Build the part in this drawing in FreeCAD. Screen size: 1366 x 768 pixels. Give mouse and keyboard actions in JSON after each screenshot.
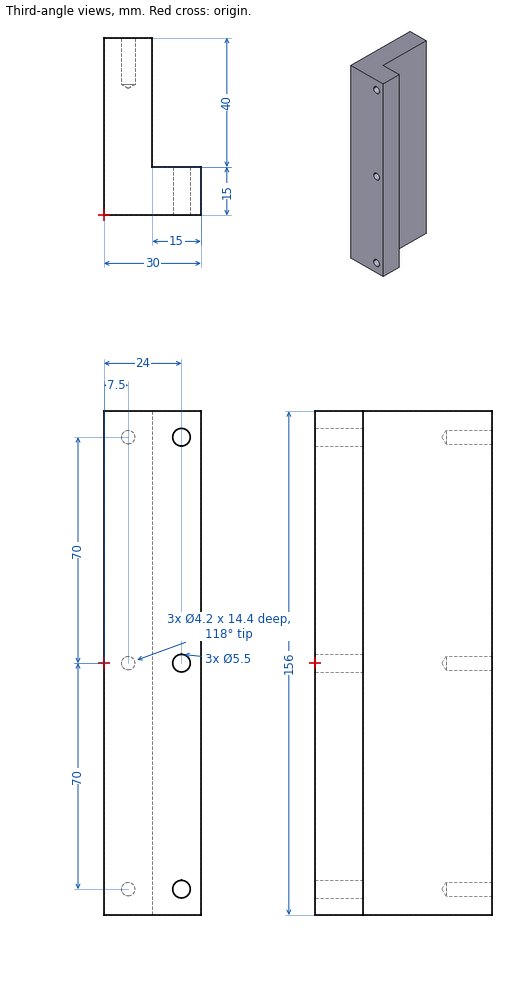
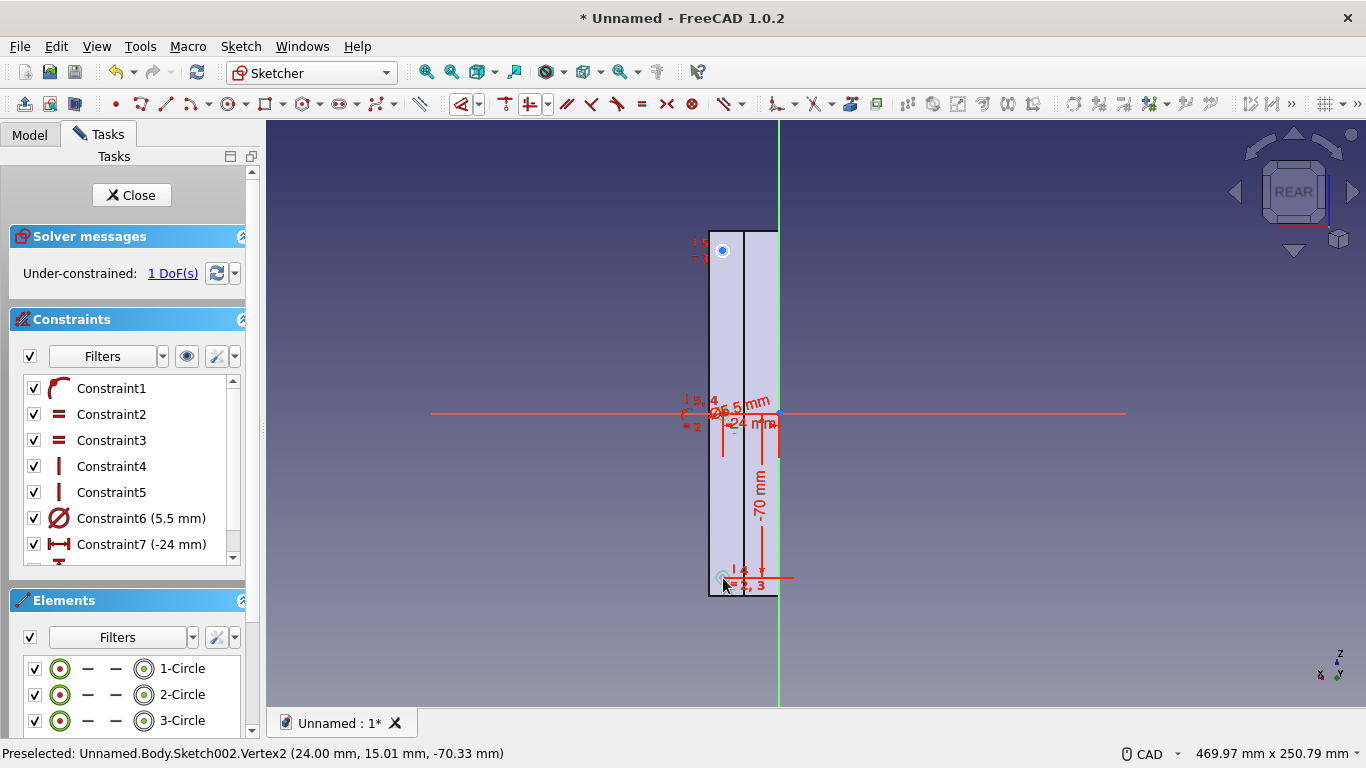
{"action": "left_click", "coordinate": [723, 251]}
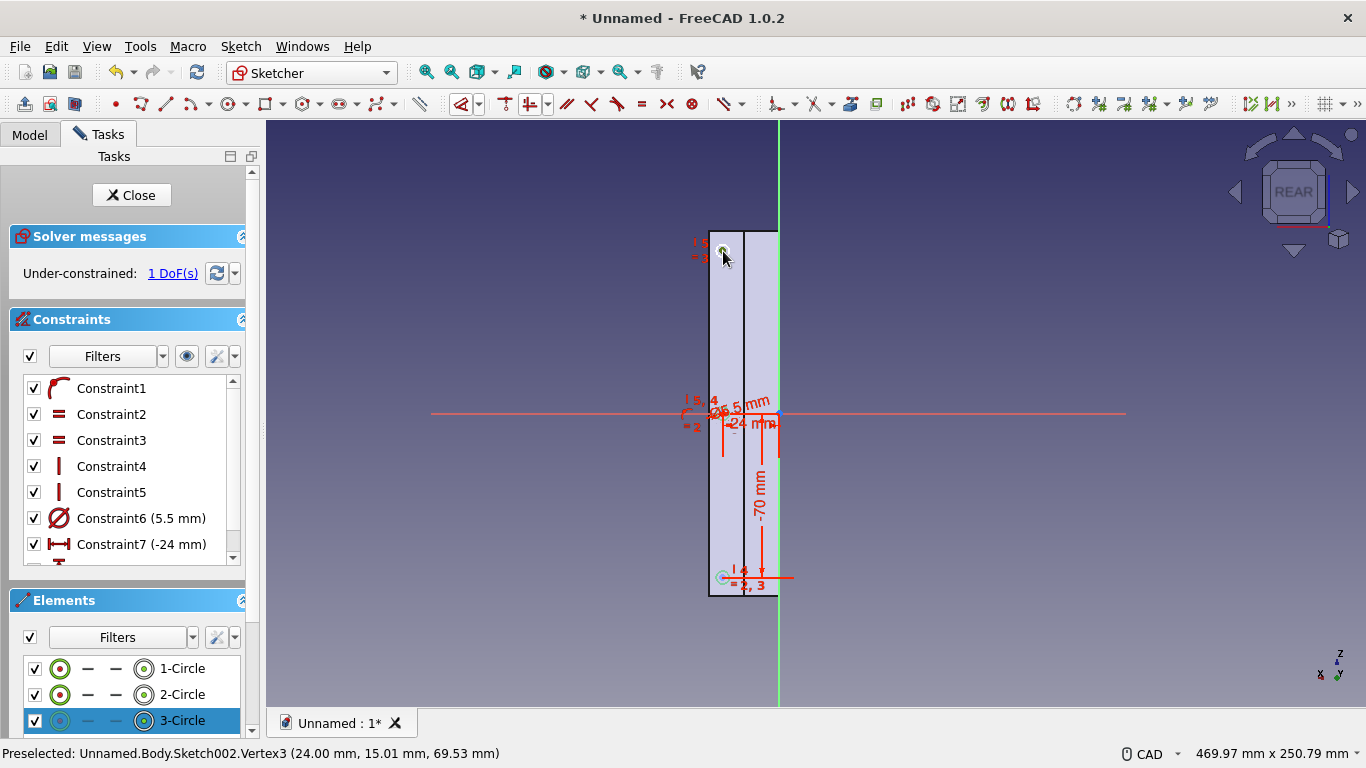
{"action": "key", "text": "i"}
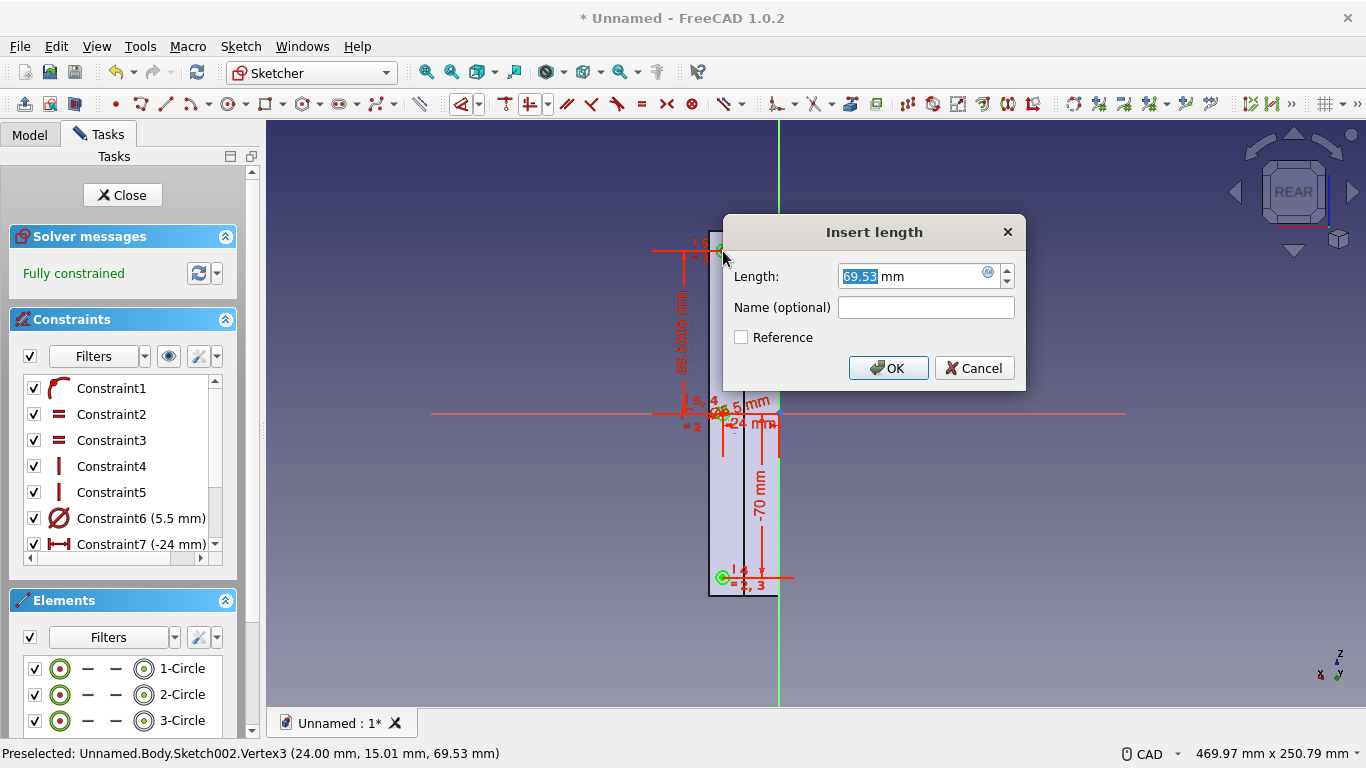
{"action": "type", "text": "70"}
{"action": "key", "text": "Return"}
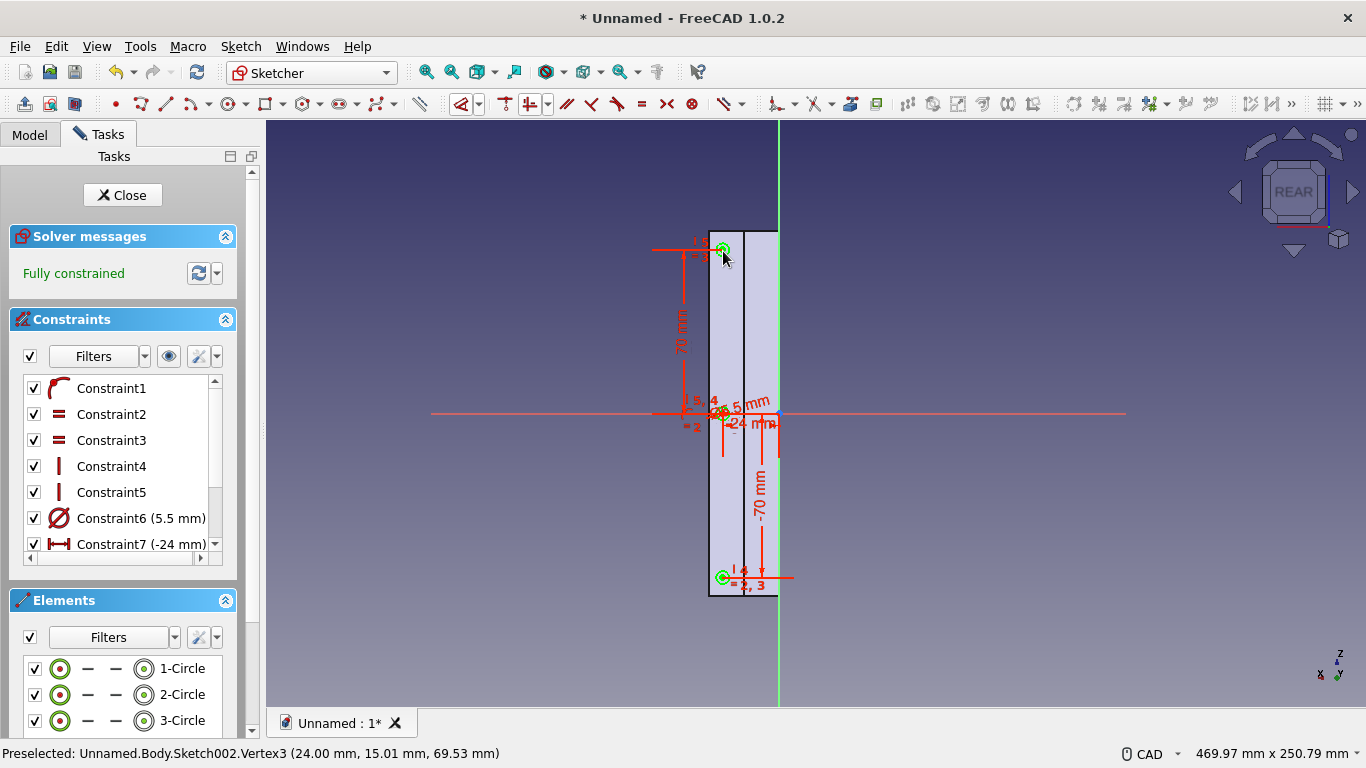
{"action": "left_click", "coordinate": [123, 195]}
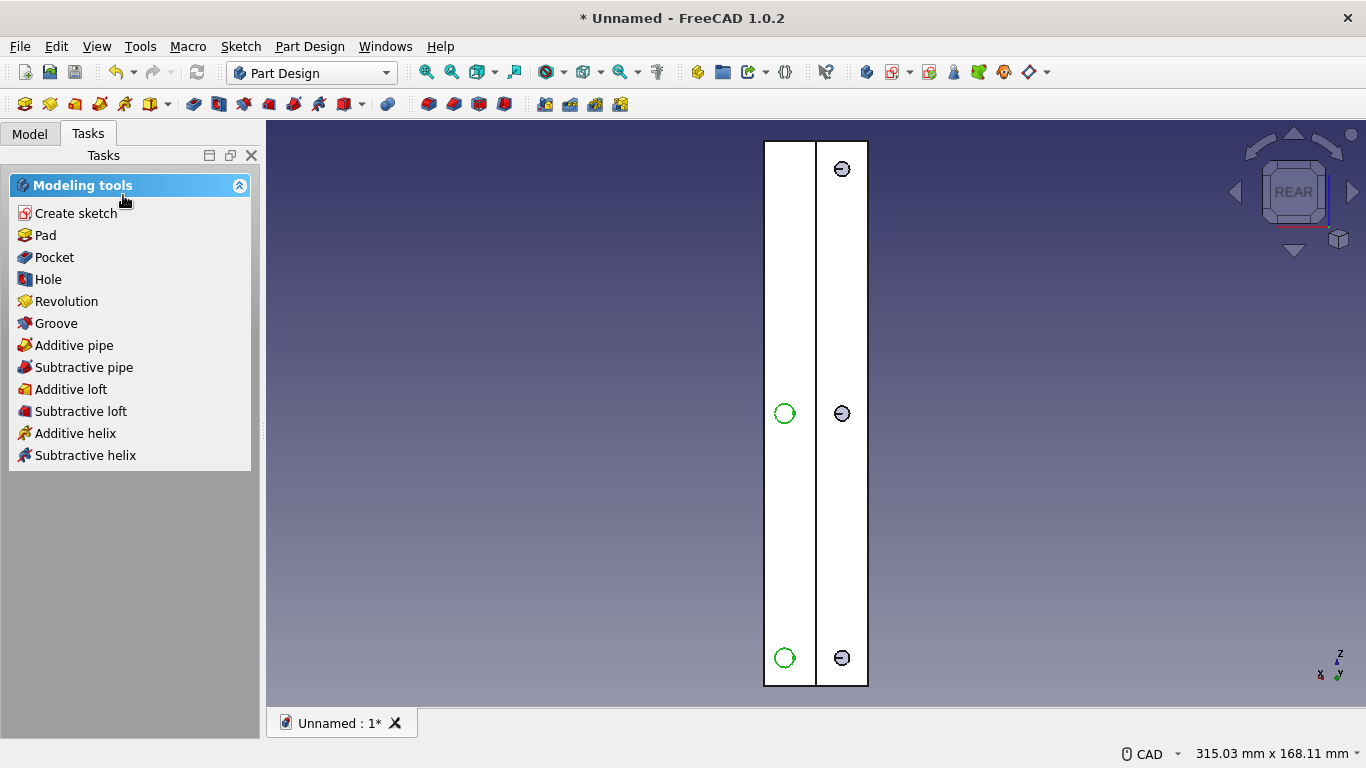
{"action": "left_click", "coordinate": [194, 104]}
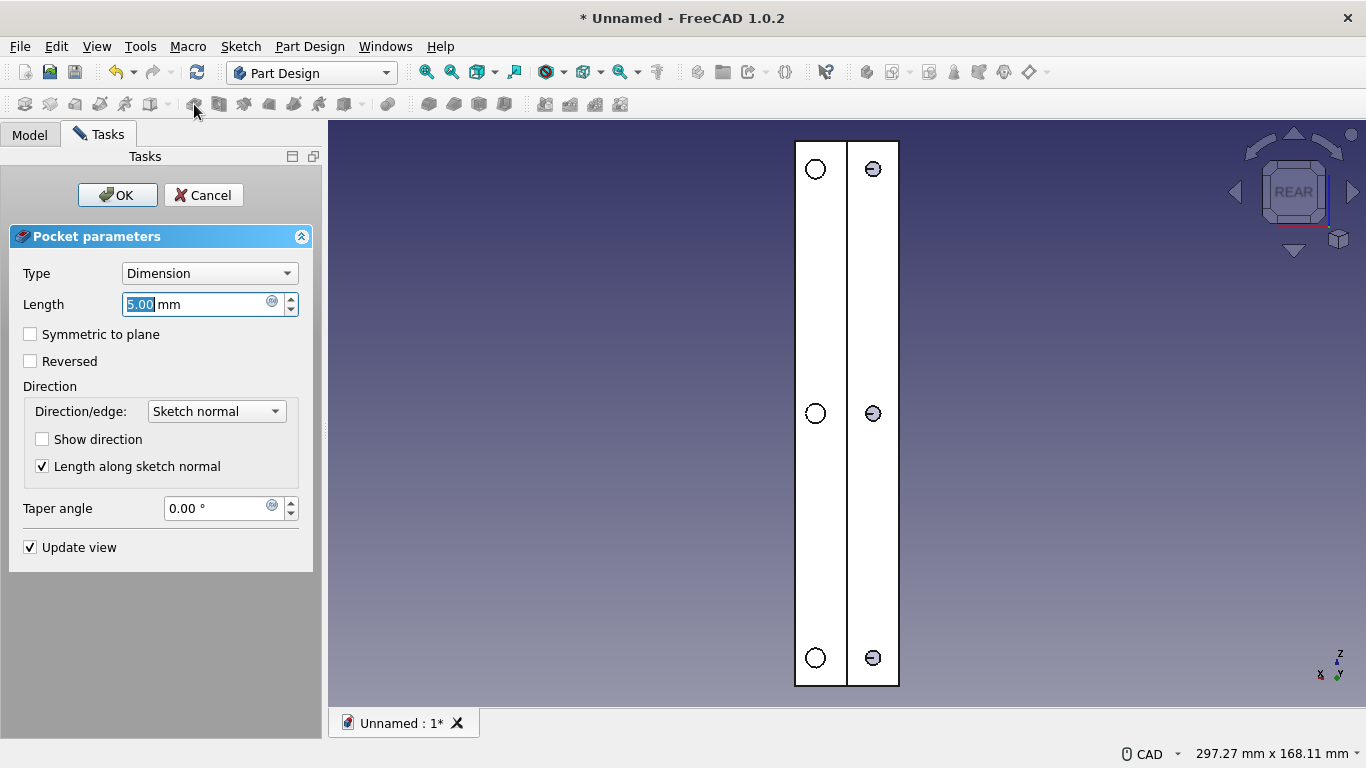
{"action": "left_click", "coordinate": [210, 274]}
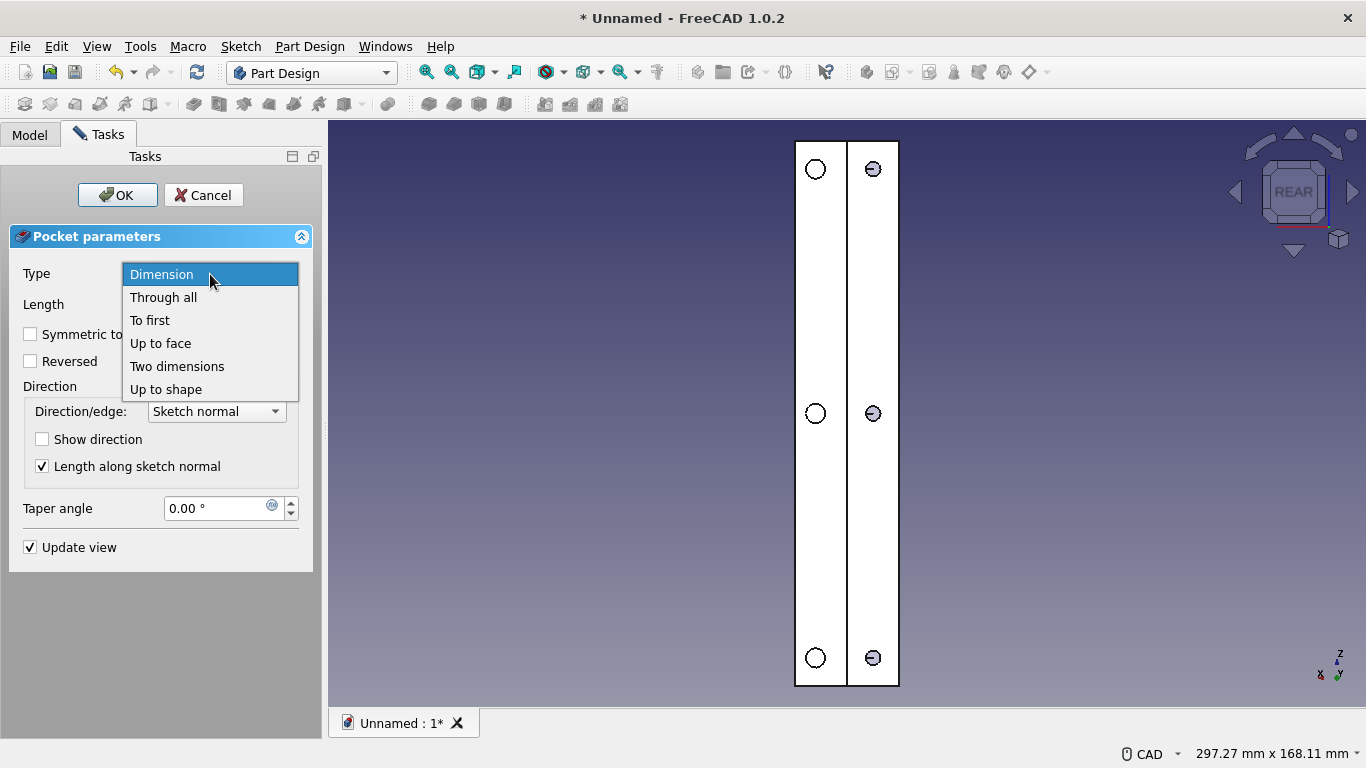
{"action": "left_click", "coordinate": [208, 298]}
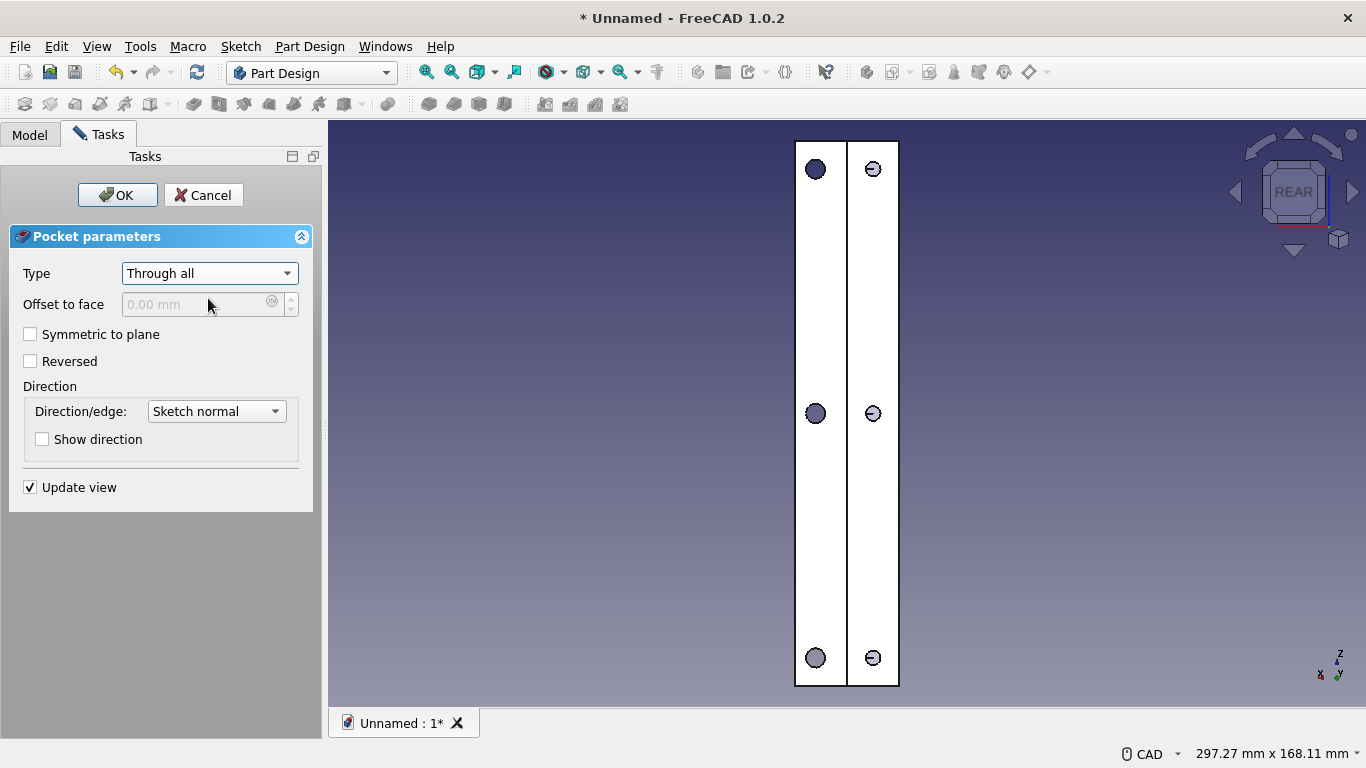
{"action": "left_click", "coordinate": [118, 195]}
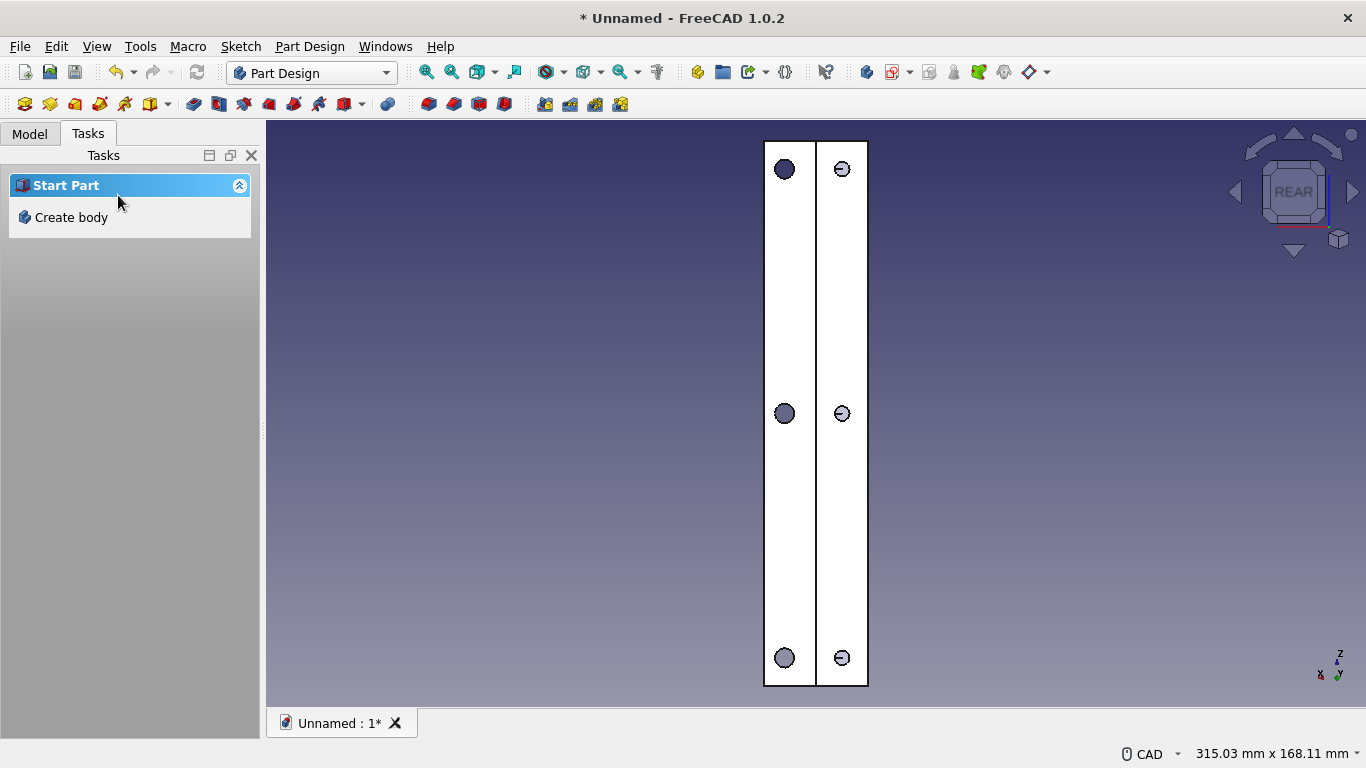
{"action": "key", "text": "0"}